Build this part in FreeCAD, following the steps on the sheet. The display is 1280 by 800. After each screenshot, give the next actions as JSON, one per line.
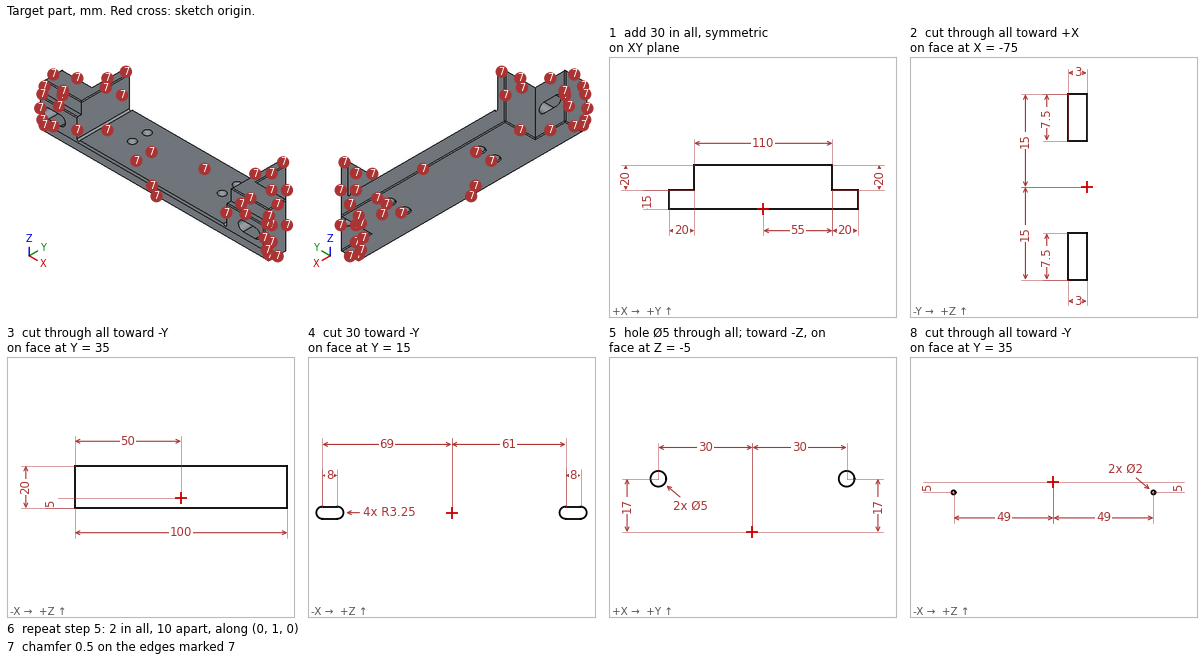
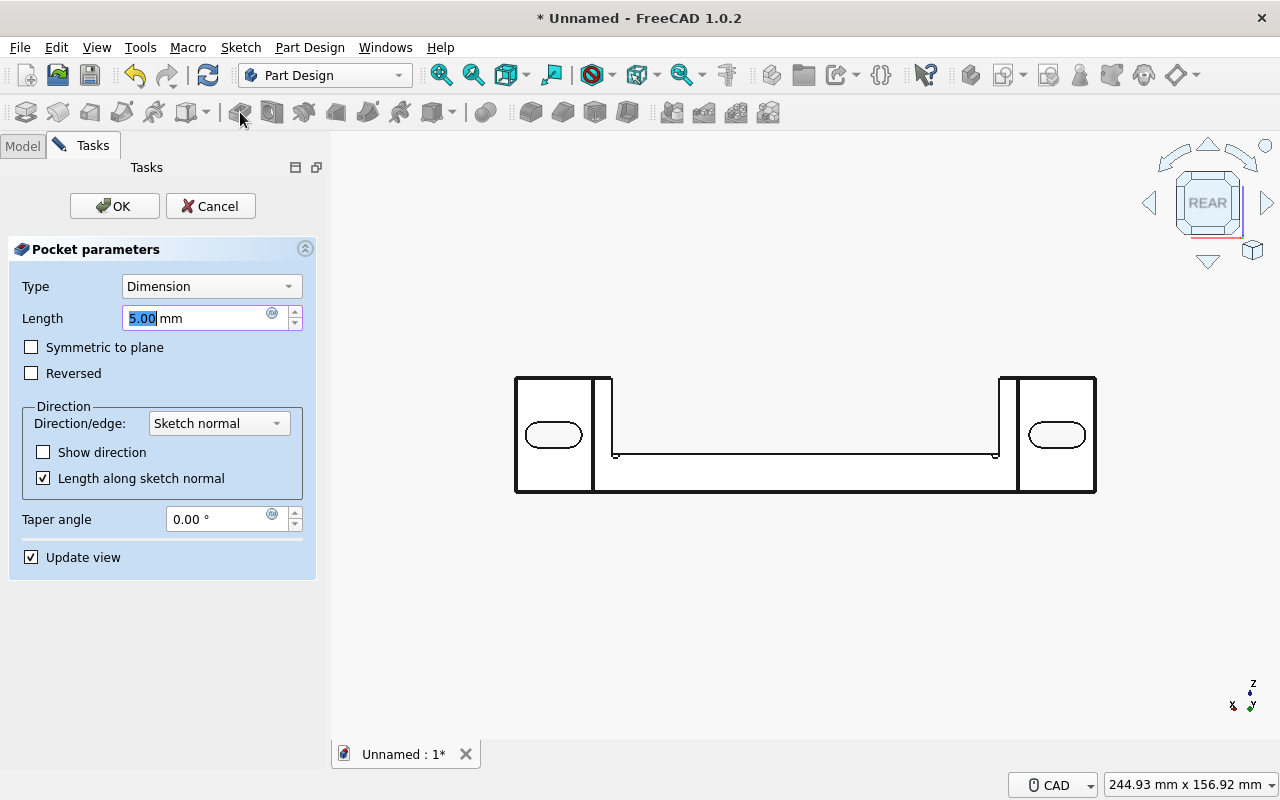
{"action": "left_click", "coordinate": [212, 286]}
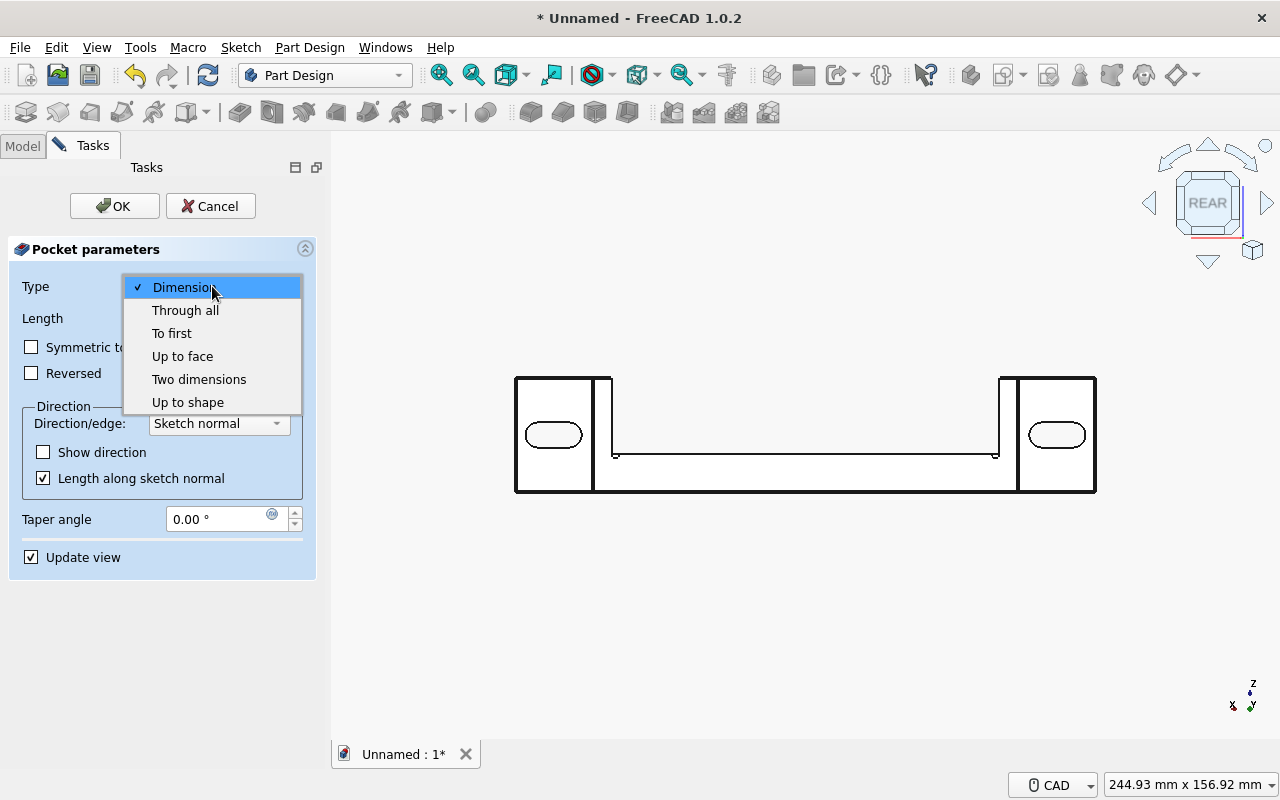
{"action": "left_click", "coordinate": [212, 310]}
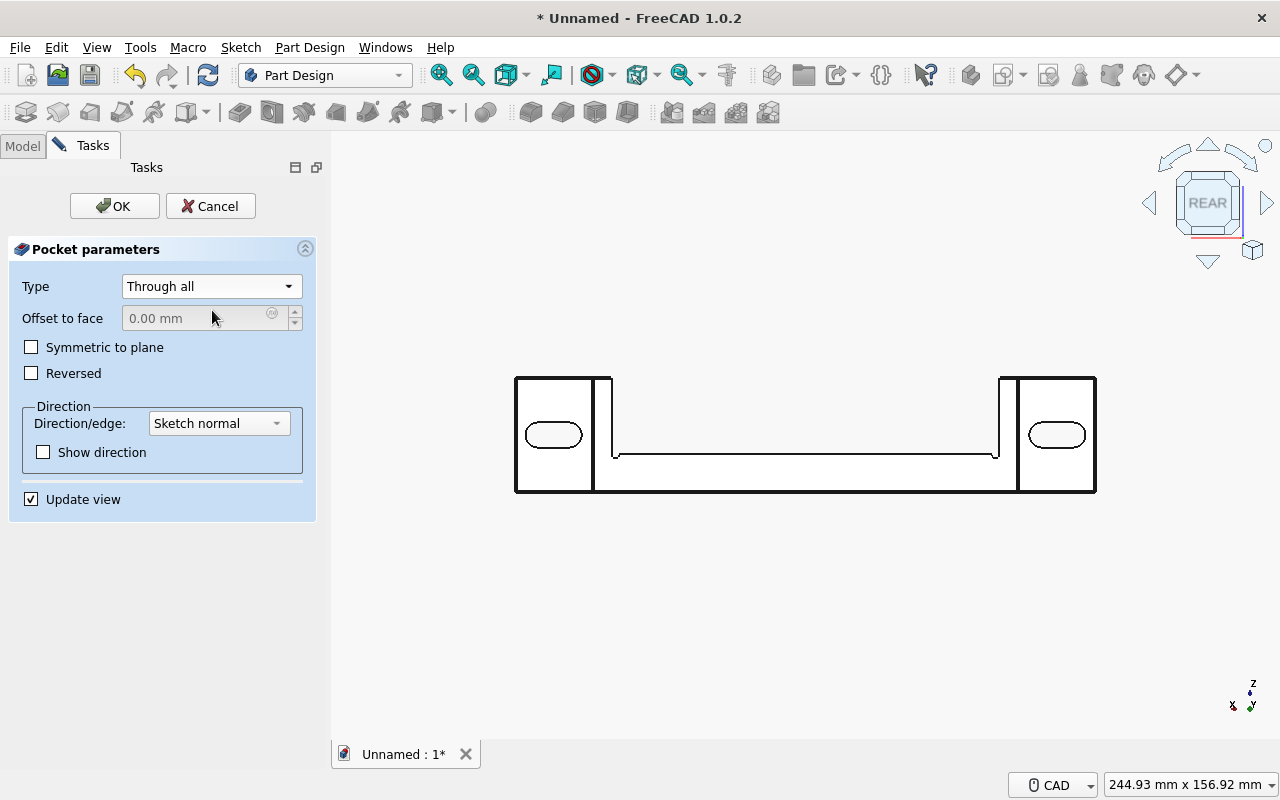
{"action": "left_click", "coordinate": [115, 206]}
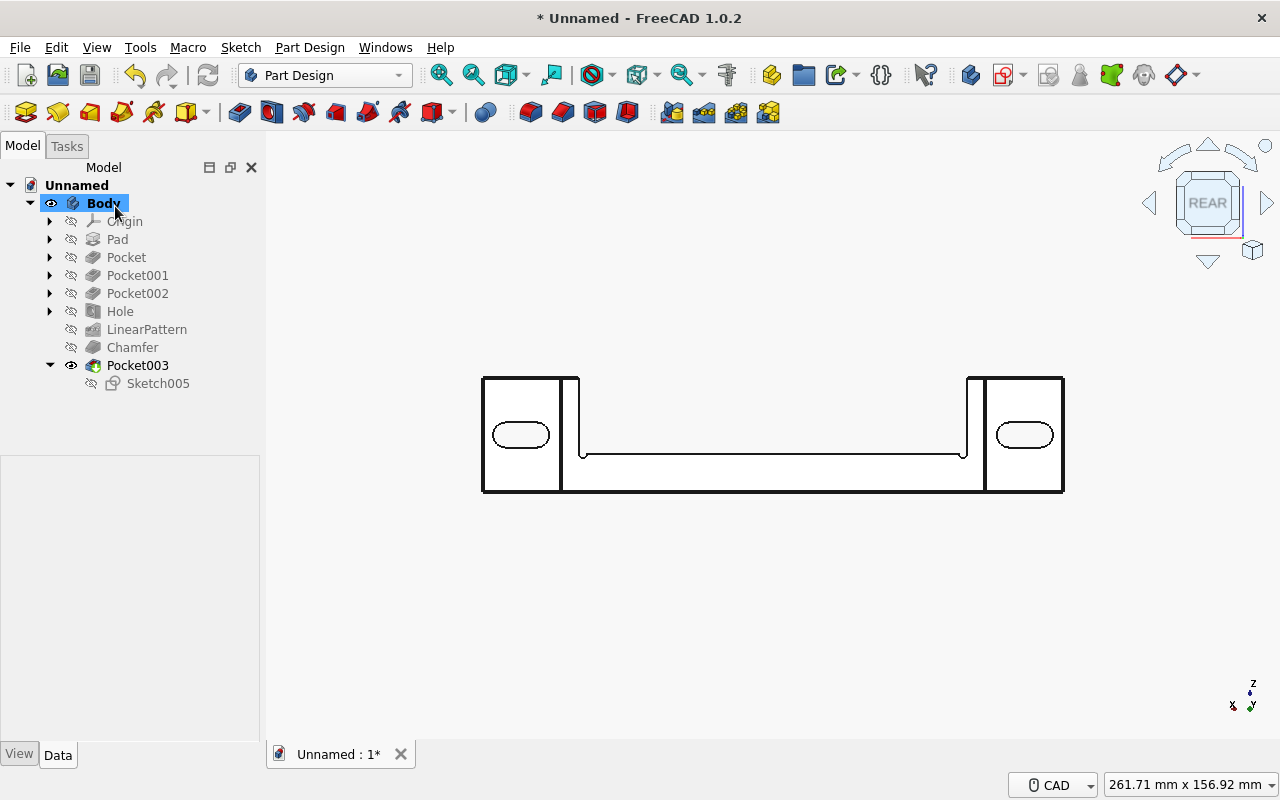
{"action": "key", "text": "0"}